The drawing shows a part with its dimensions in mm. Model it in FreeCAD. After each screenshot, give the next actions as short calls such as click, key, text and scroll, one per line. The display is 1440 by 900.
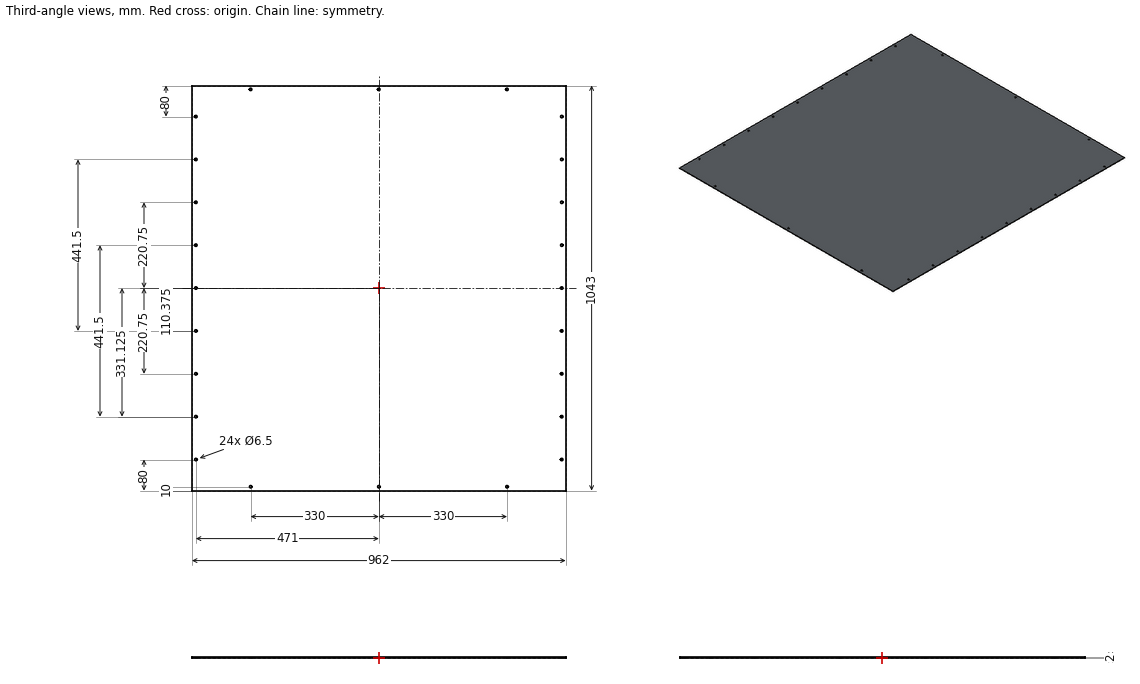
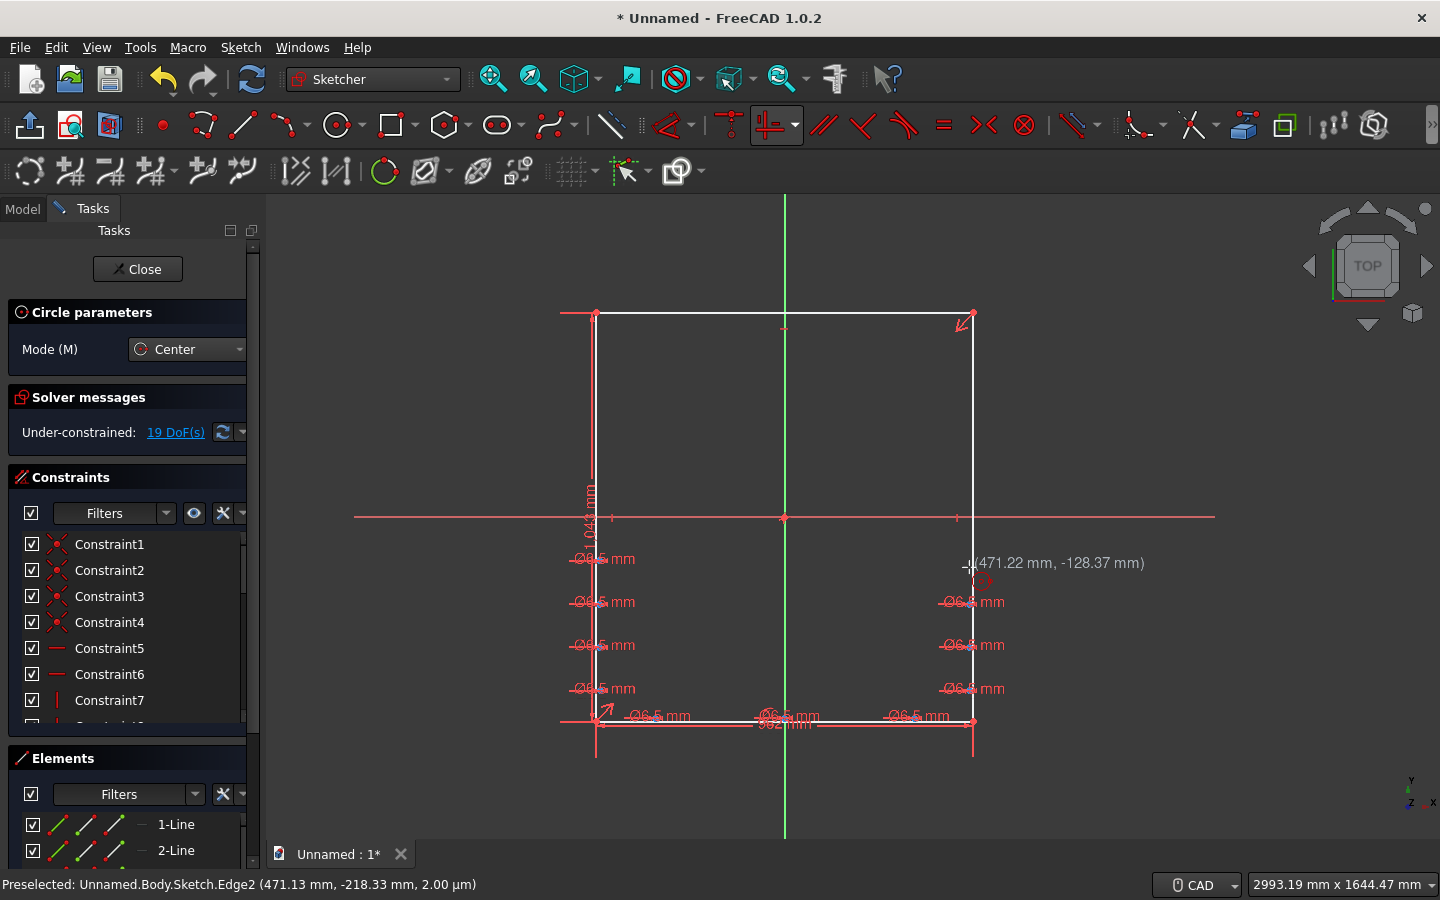
scroll(969, 561, up, 7)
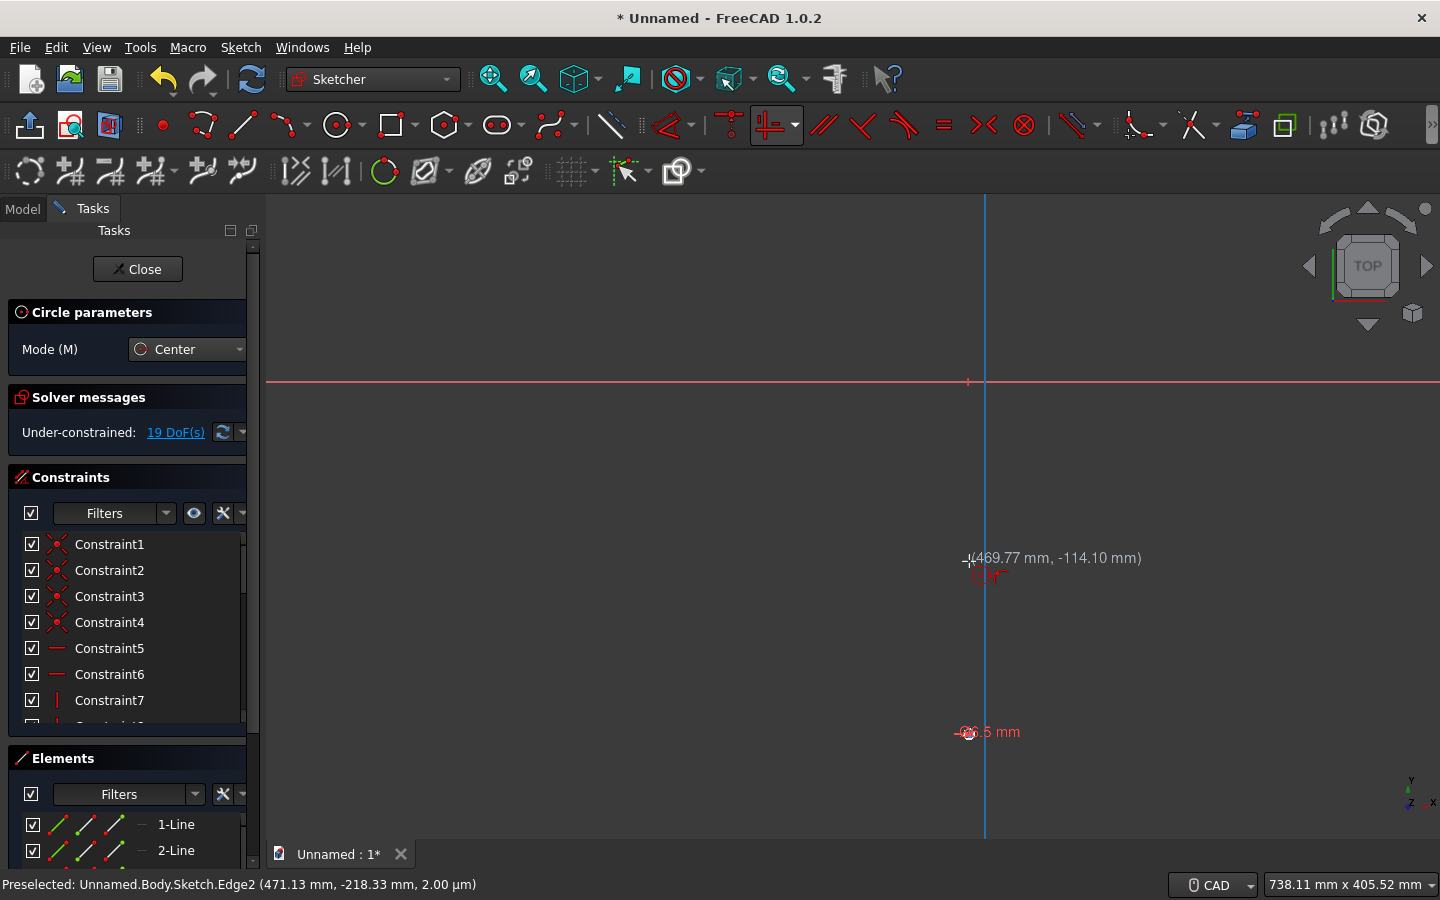
click(969, 557)
move(965, 554)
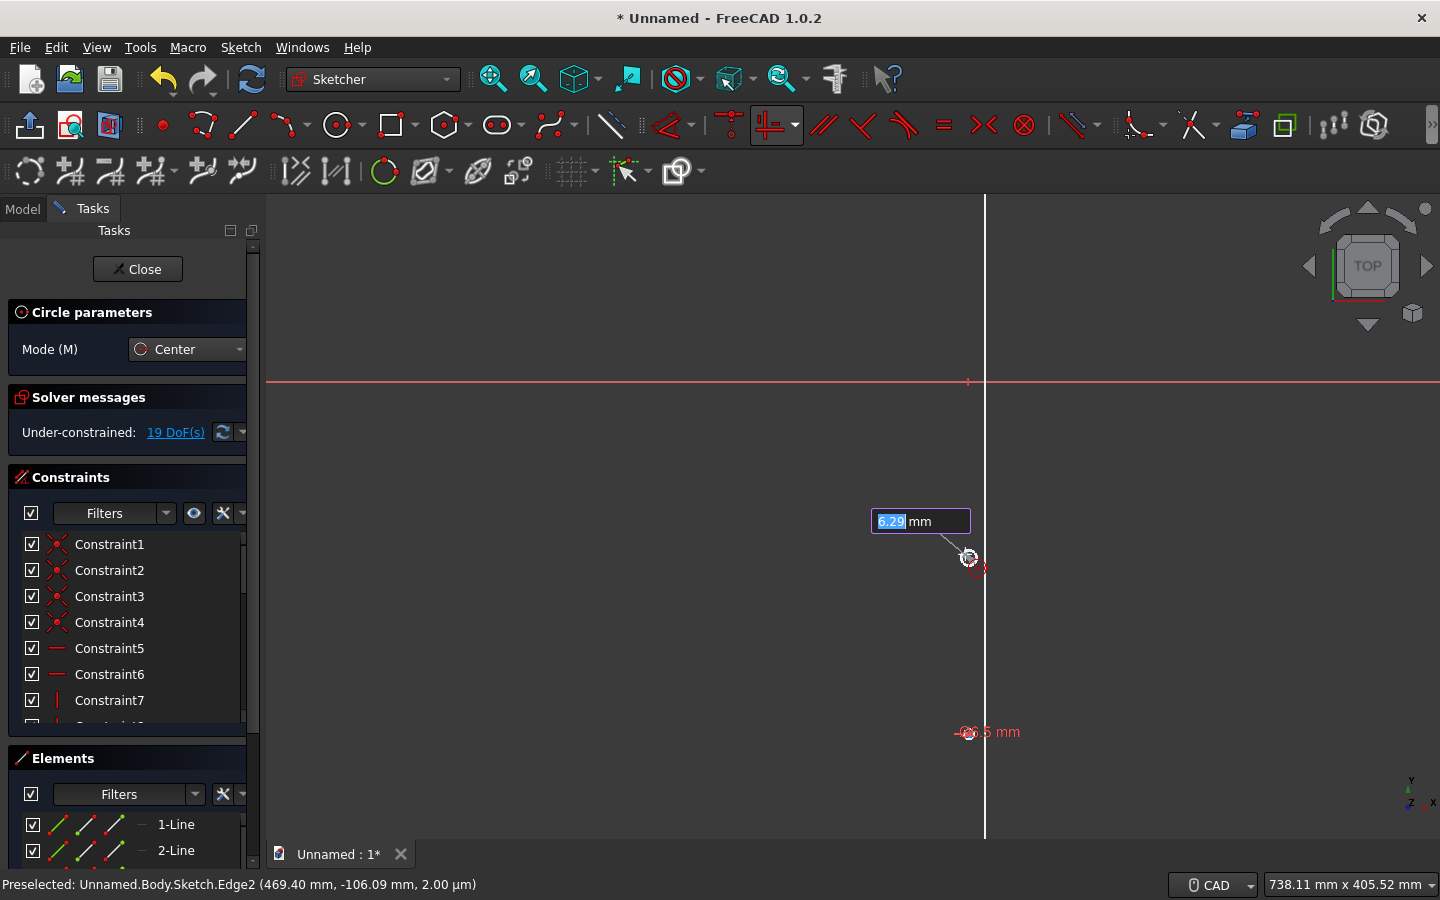
text(6.5)
key(Return)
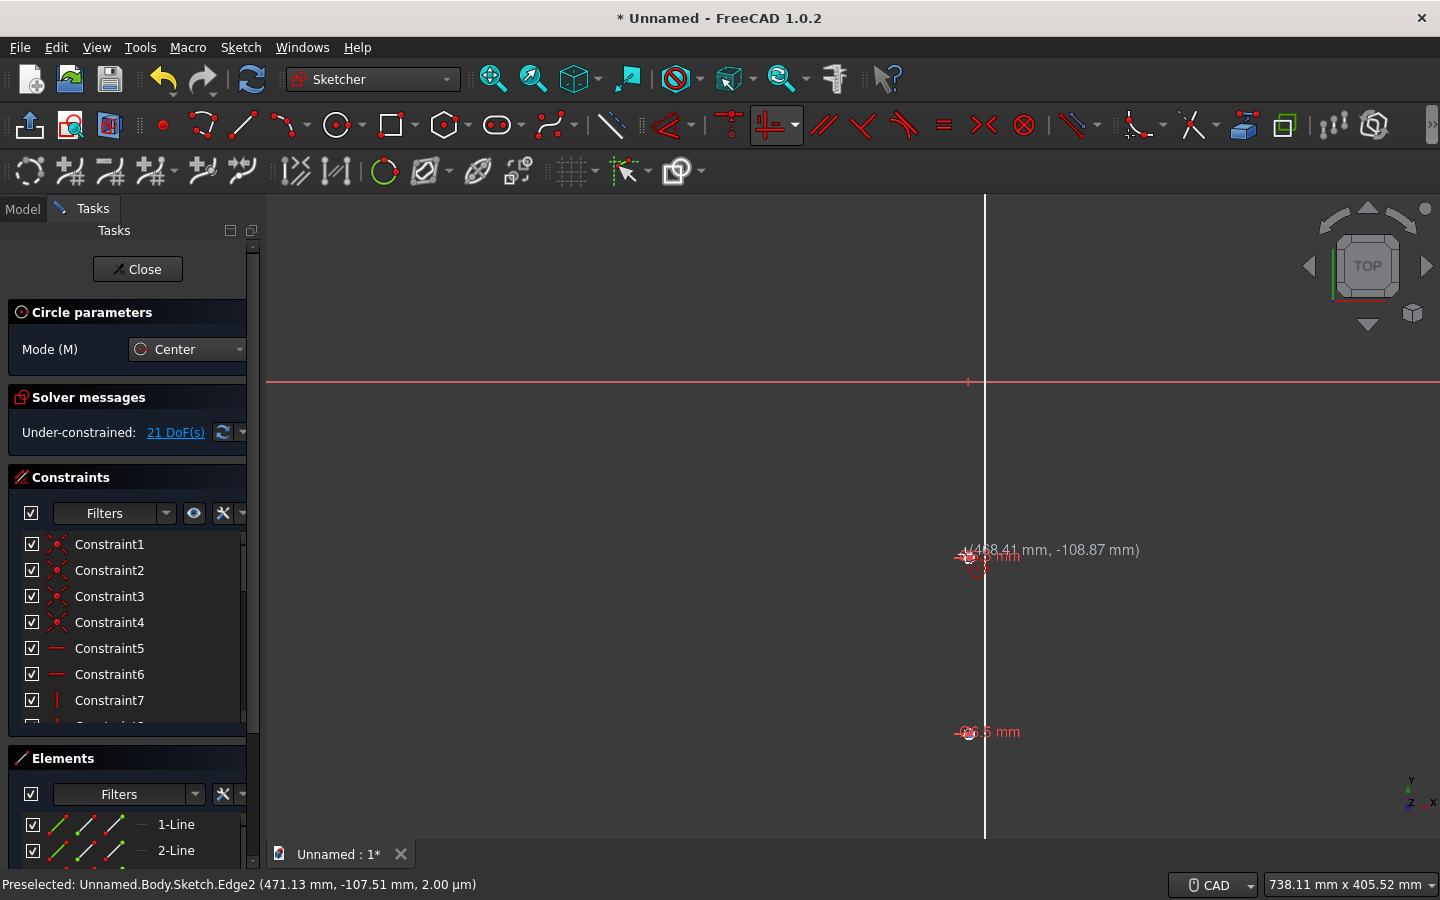
scroll(969, 561, down, 7)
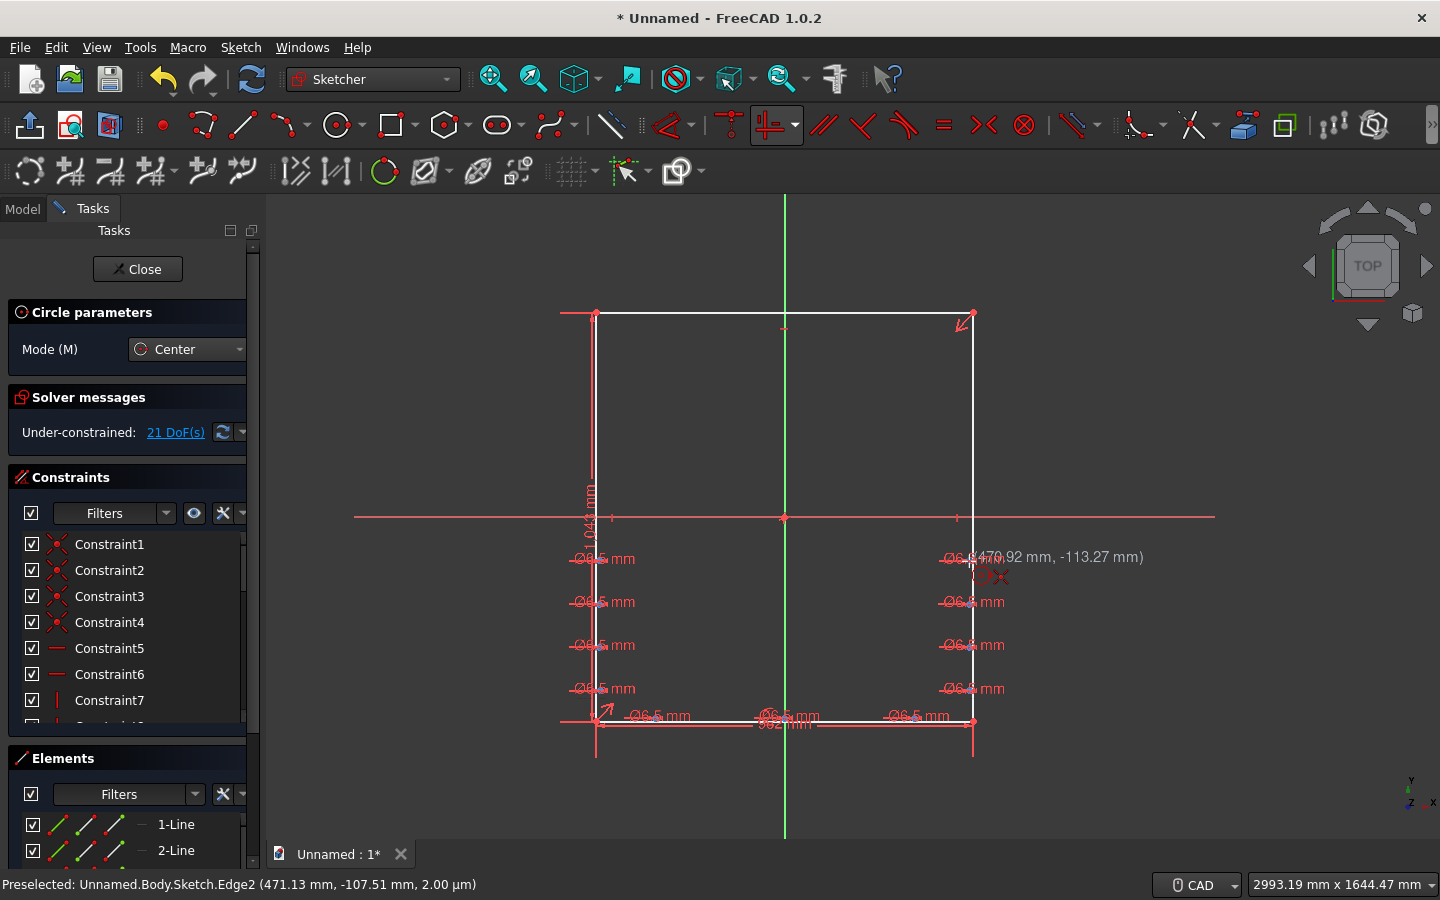
scroll(600, 517, up, 15)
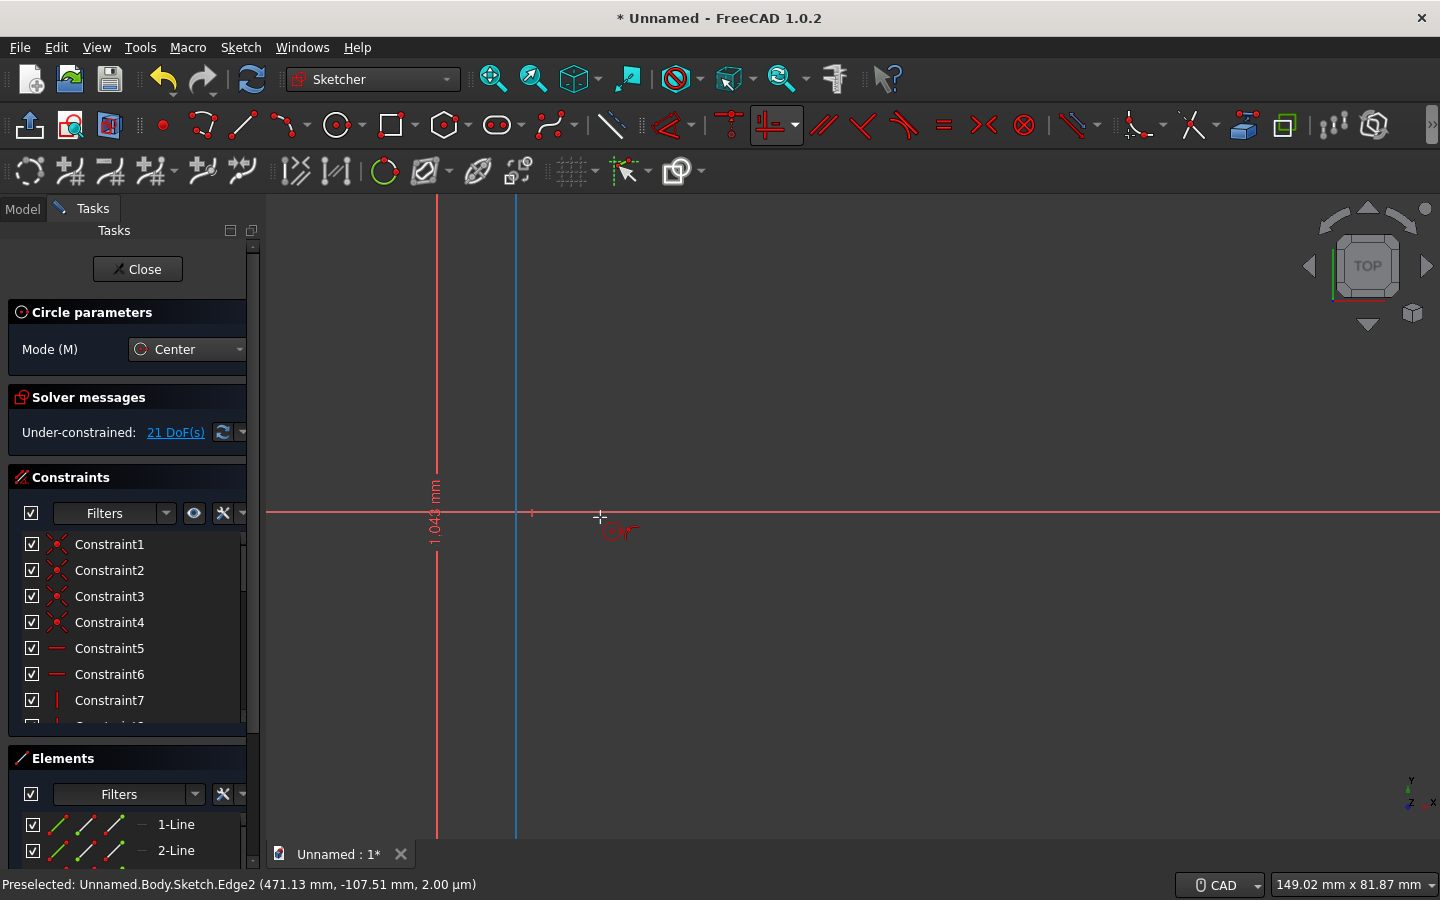
scroll(600, 517, down, 15)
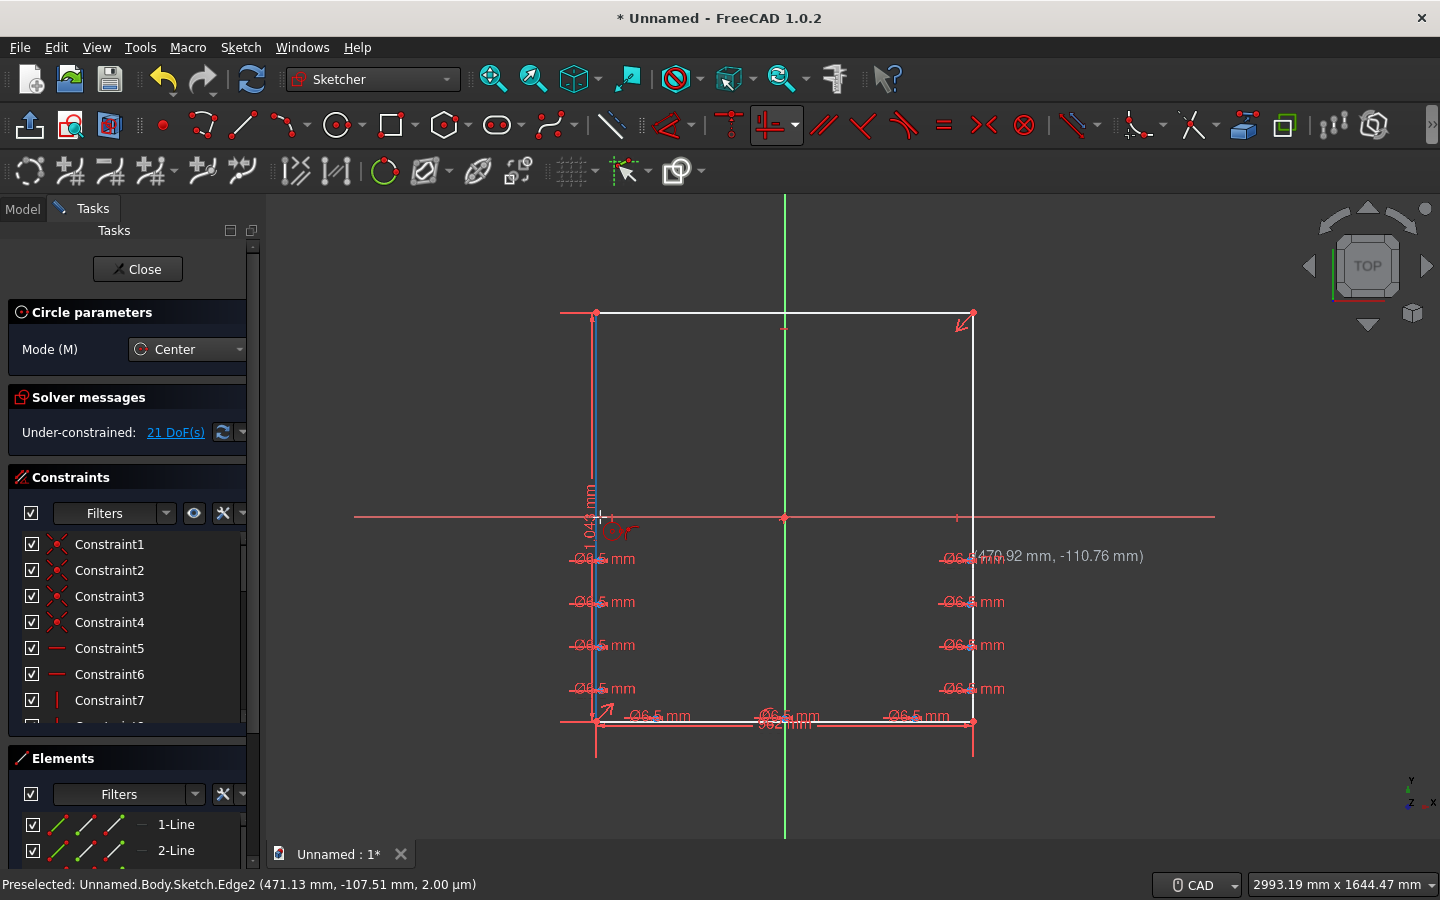
scroll(600, 517, up, 7)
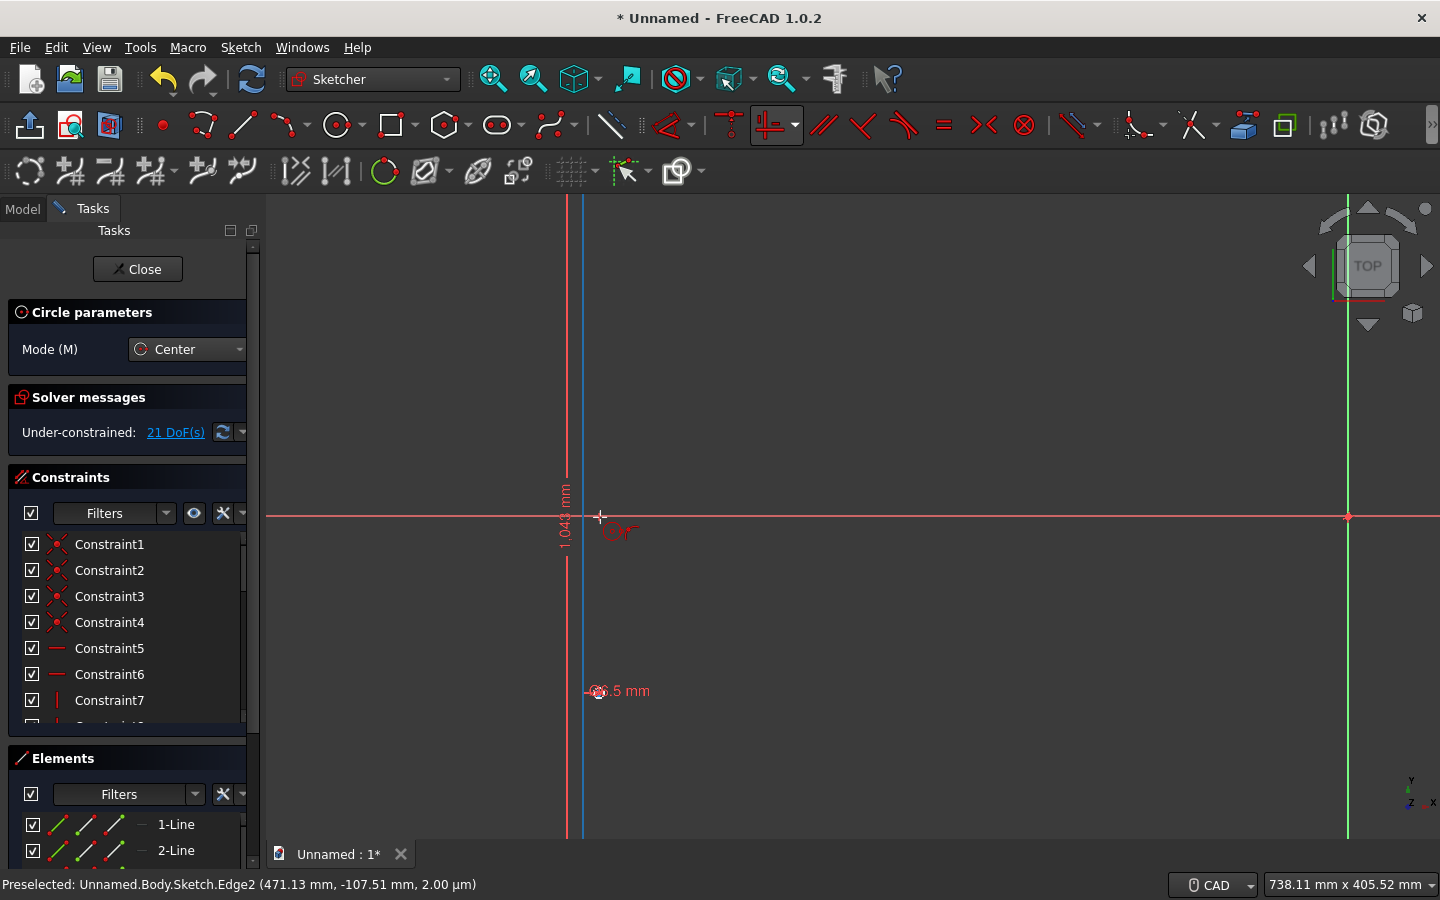
click(599, 516)